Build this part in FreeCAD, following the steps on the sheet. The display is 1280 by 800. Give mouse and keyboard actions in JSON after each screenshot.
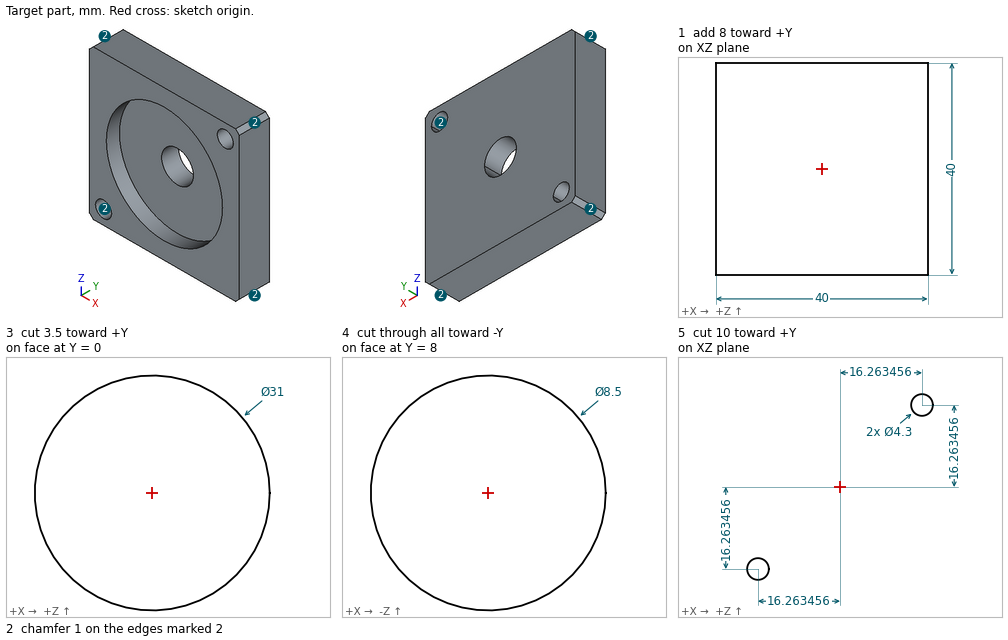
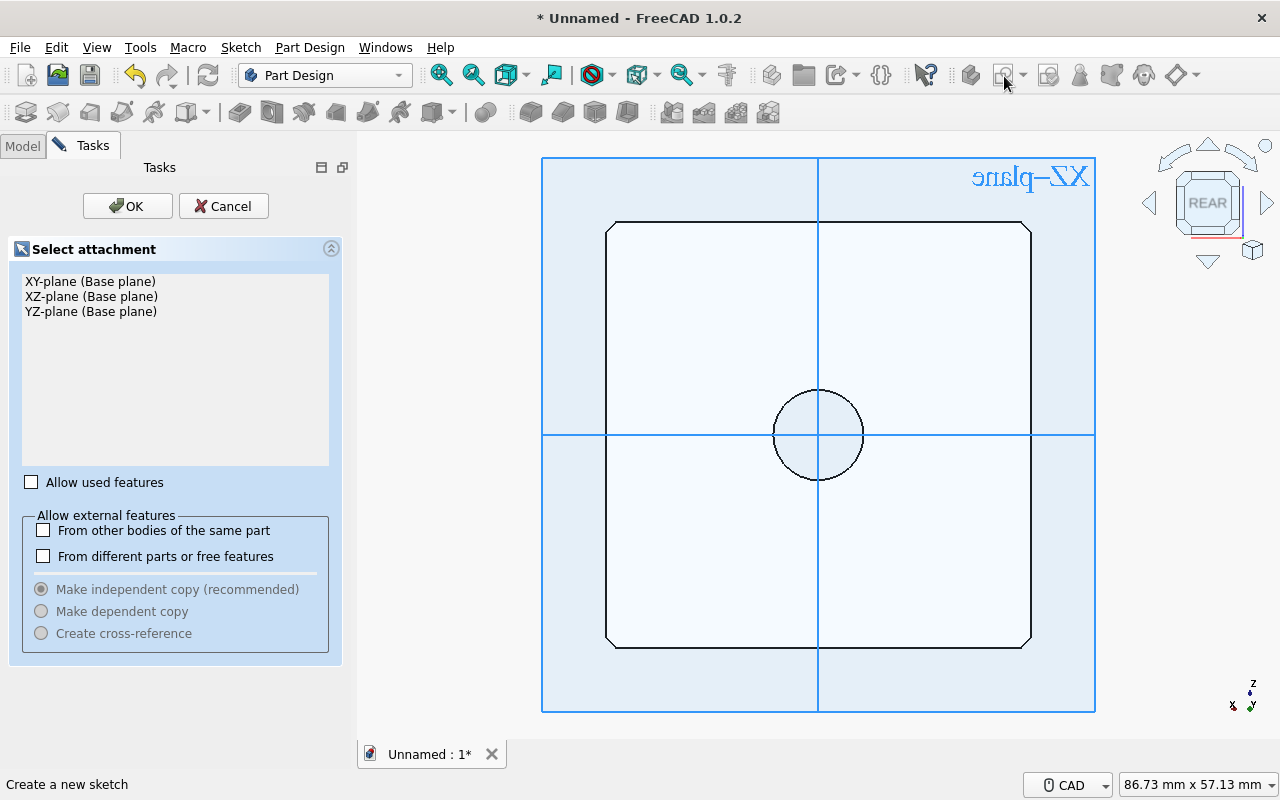
{"action": "left_click", "coordinate": [82, 296]}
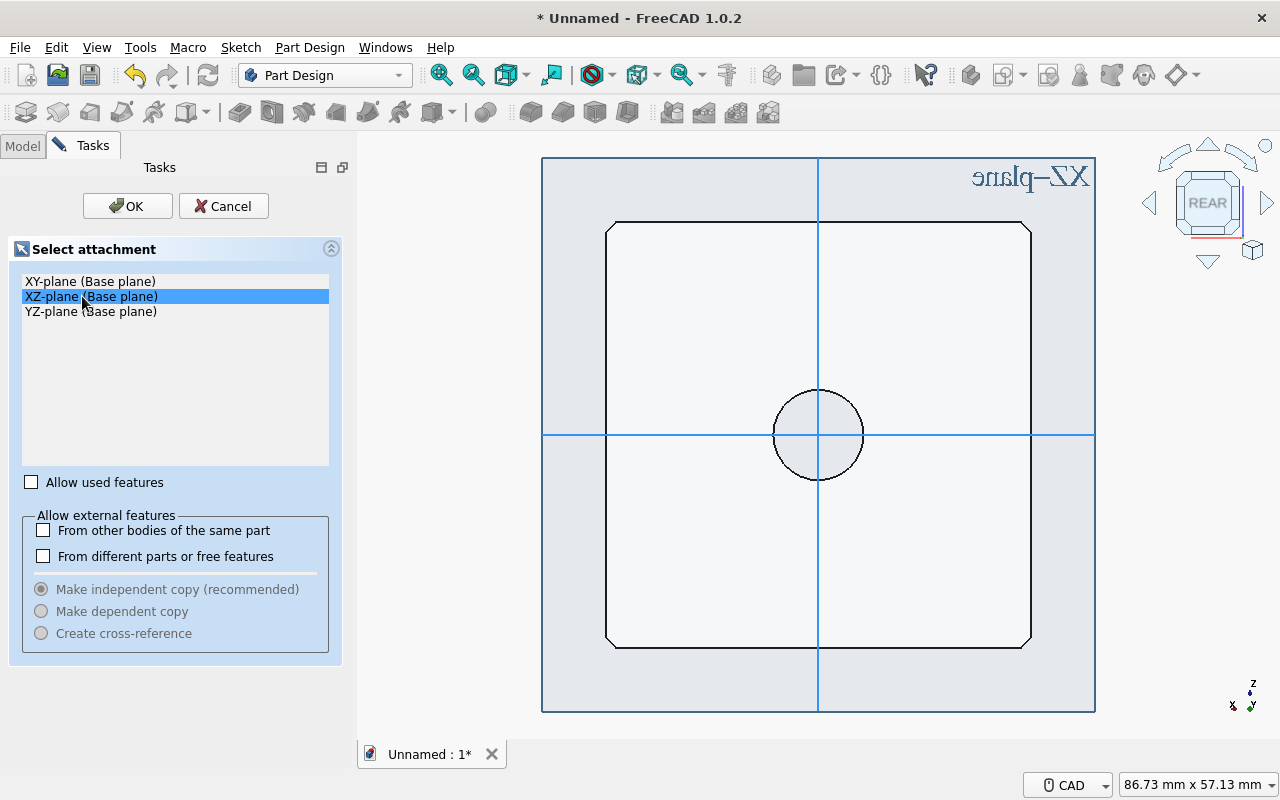
{"action": "left_click", "coordinate": [128, 206]}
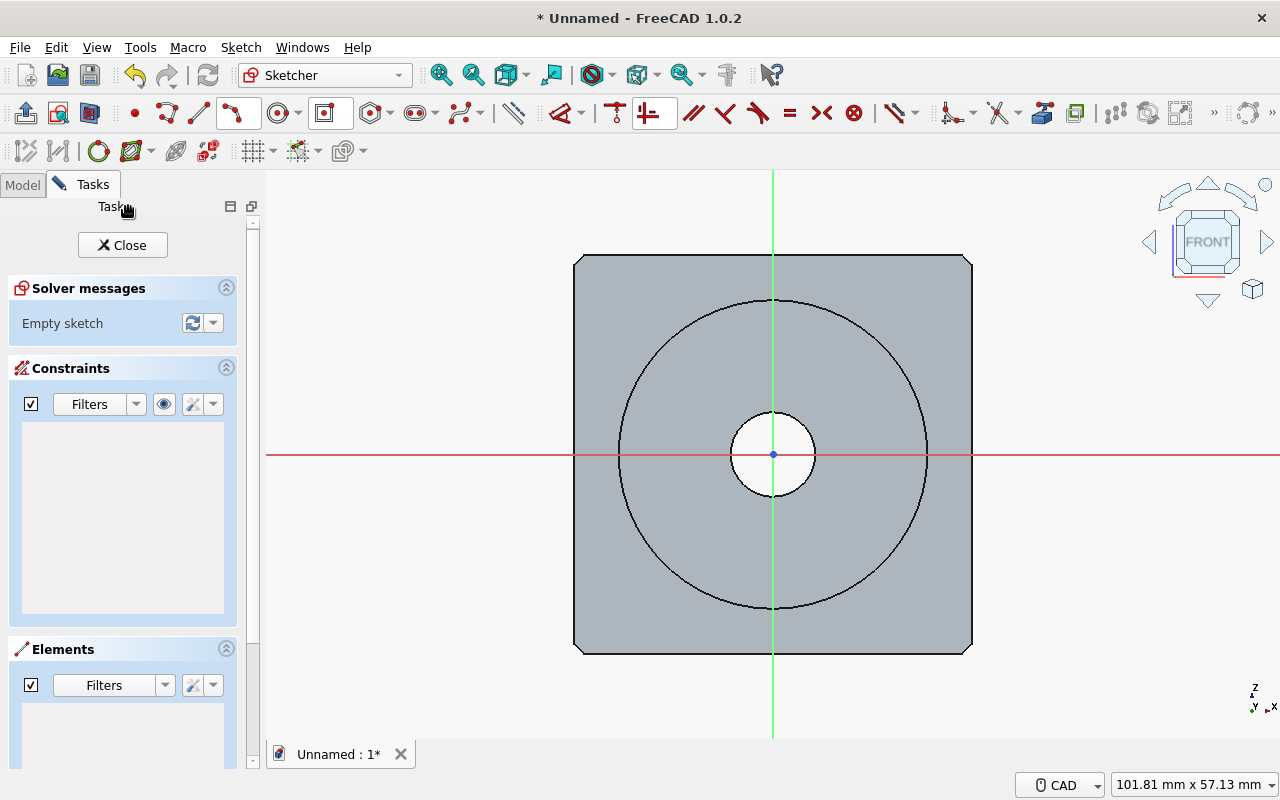
{"action": "left_click", "coordinate": [278, 114]}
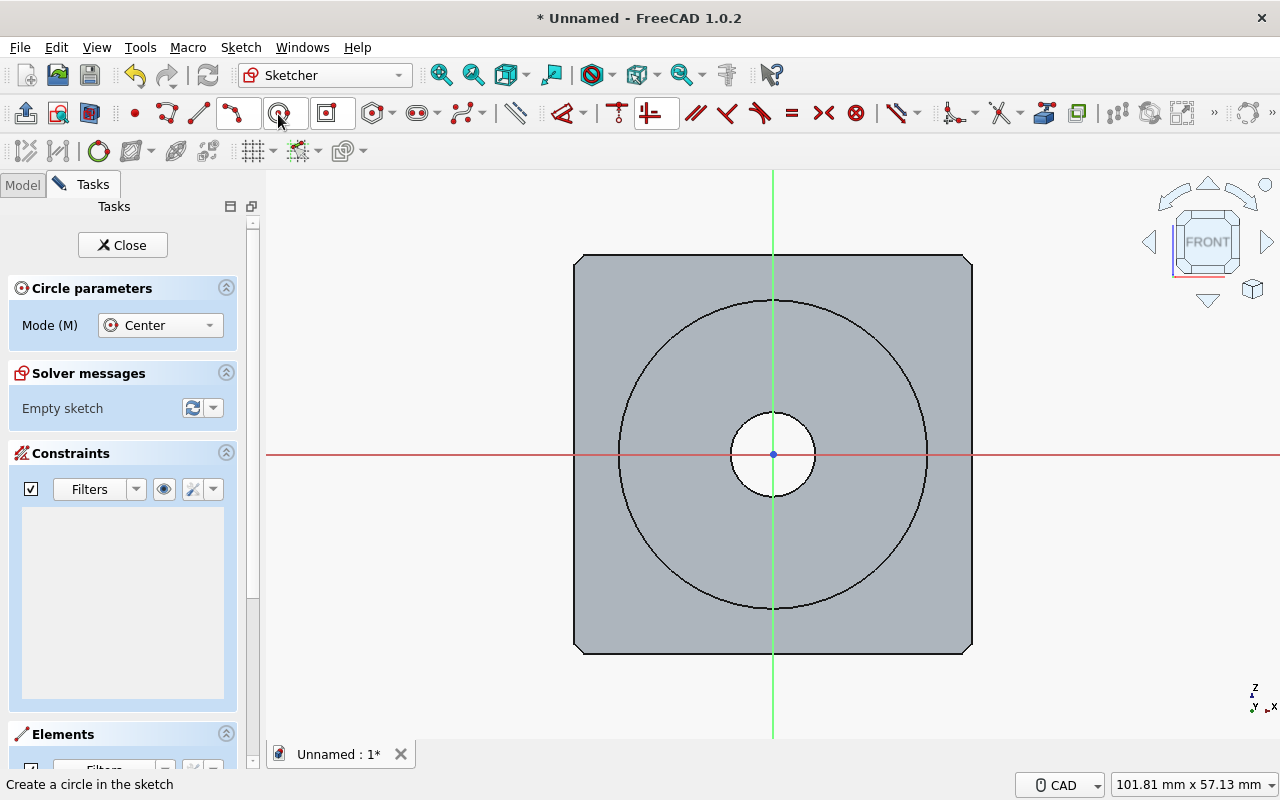
{"action": "left_click", "coordinate": [935, 293]}
{"action": "left_click", "coordinate": [950, 277]}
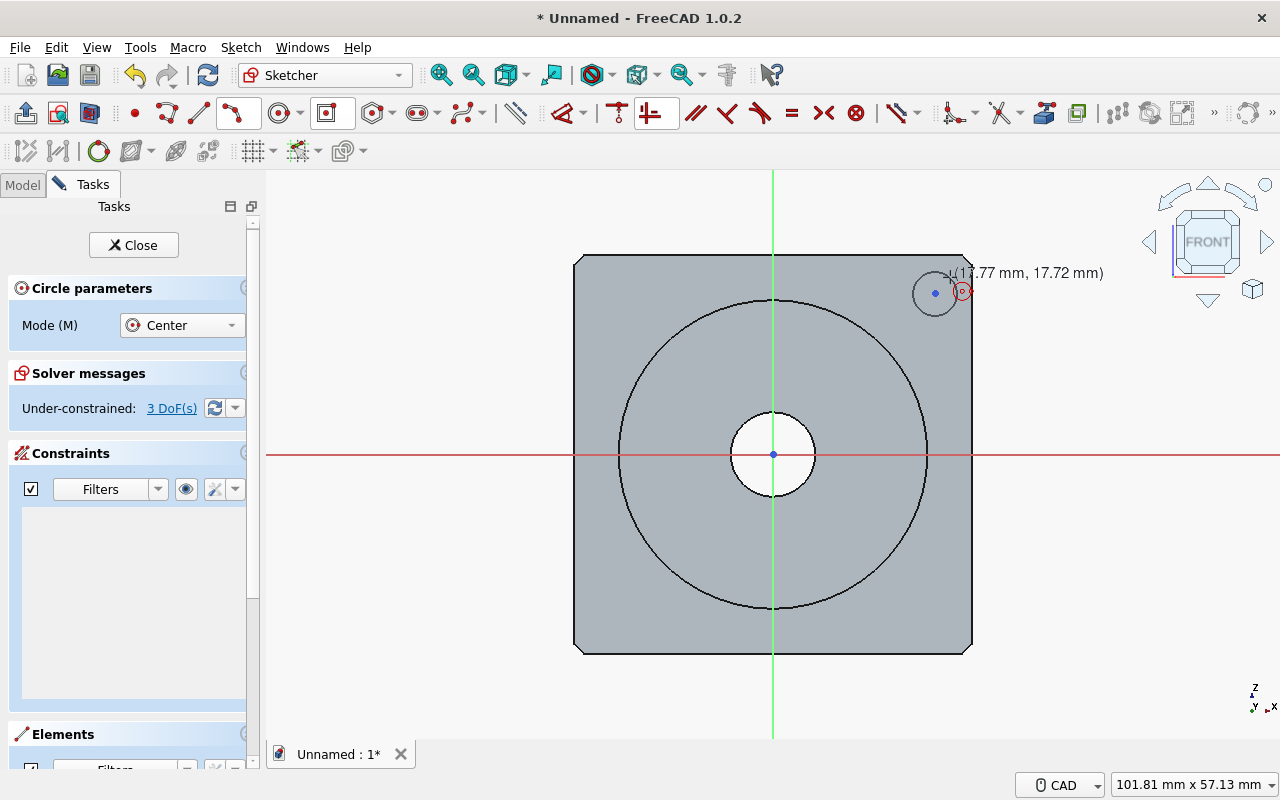
{"action": "left_click", "coordinate": [611, 616]}
{"action": "left_click", "coordinate": [626, 601]}
{"action": "key", "text": "Escape"}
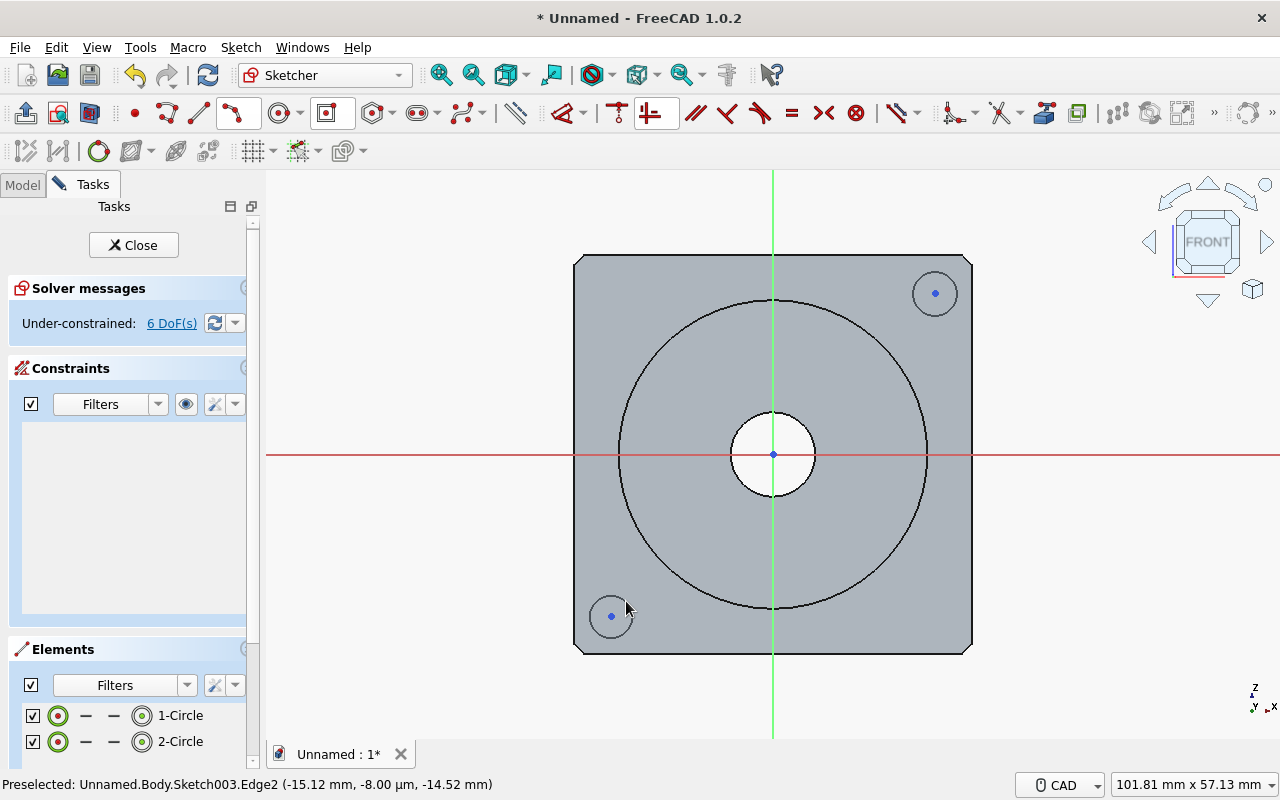
{"action": "left_click", "coordinate": [950, 278]}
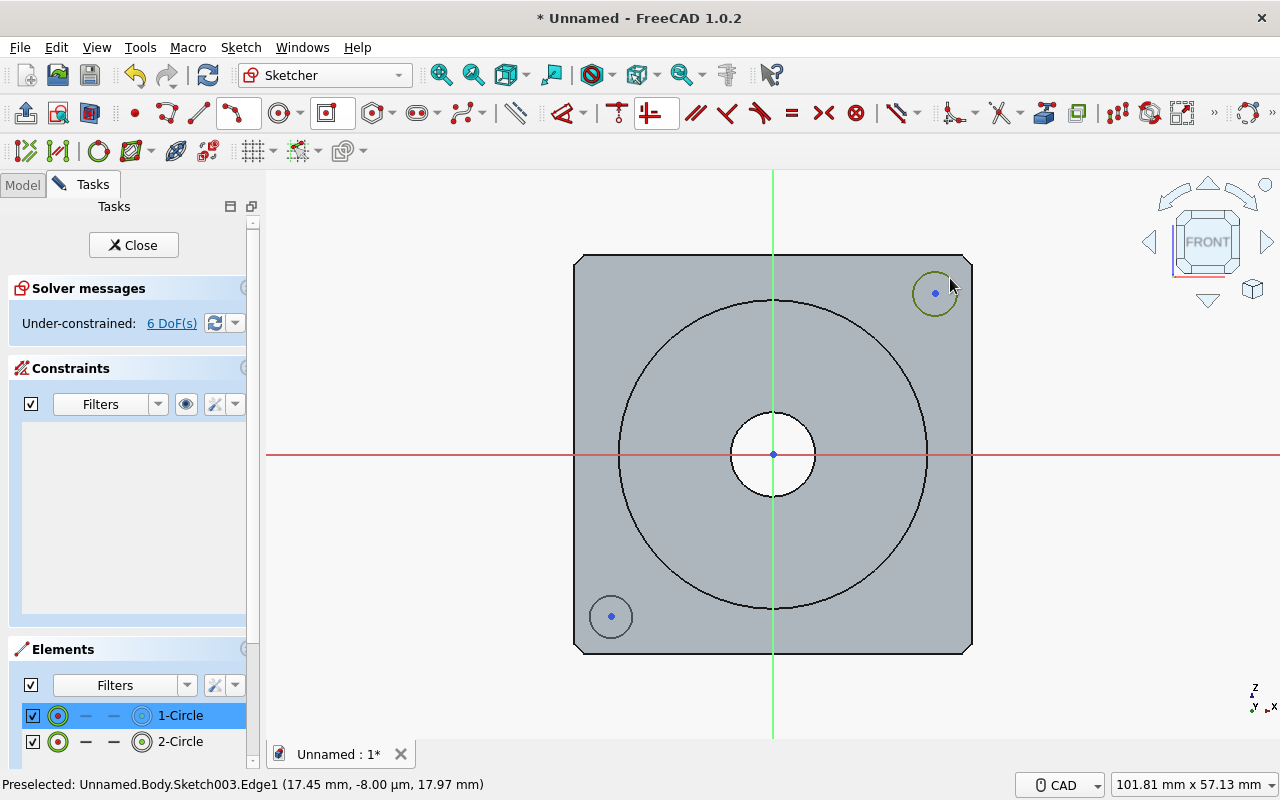
{"action": "left_click", "coordinate": [626, 602]}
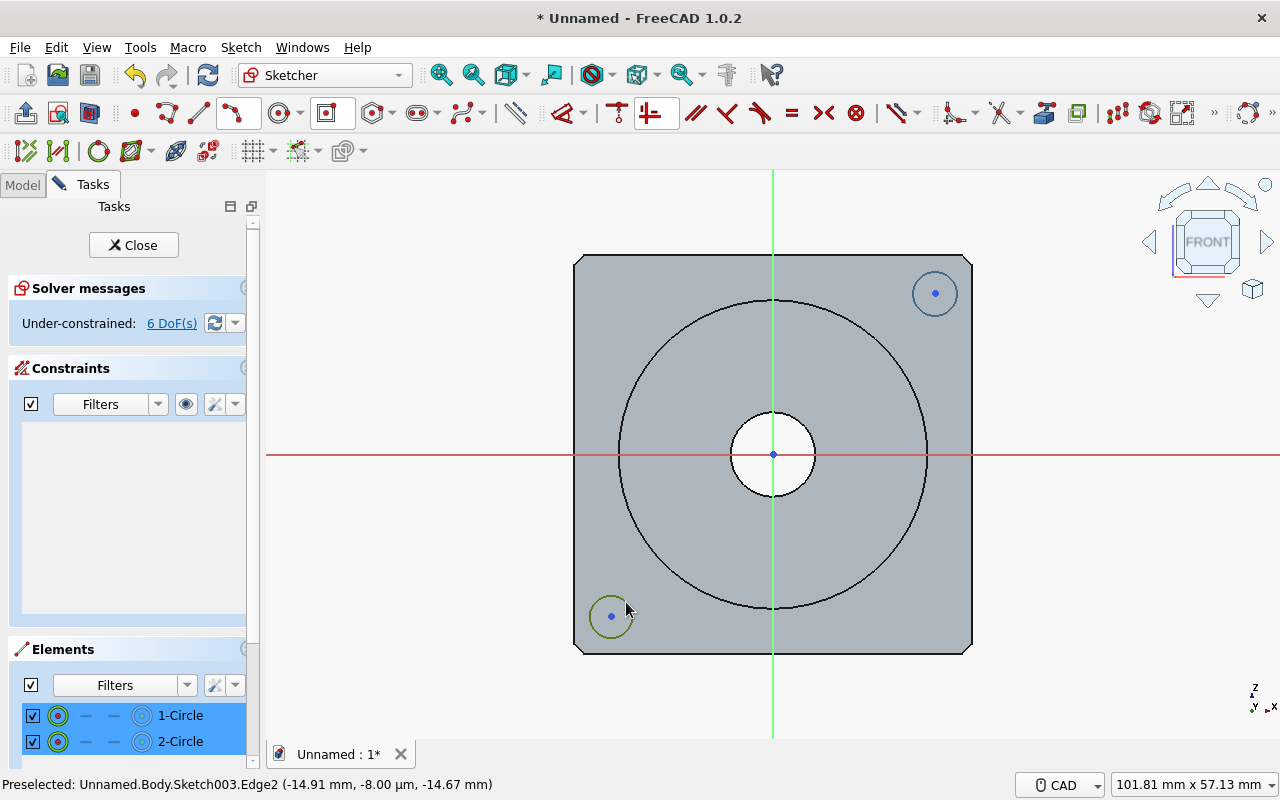
{"action": "left_click", "coordinate": [792, 114]}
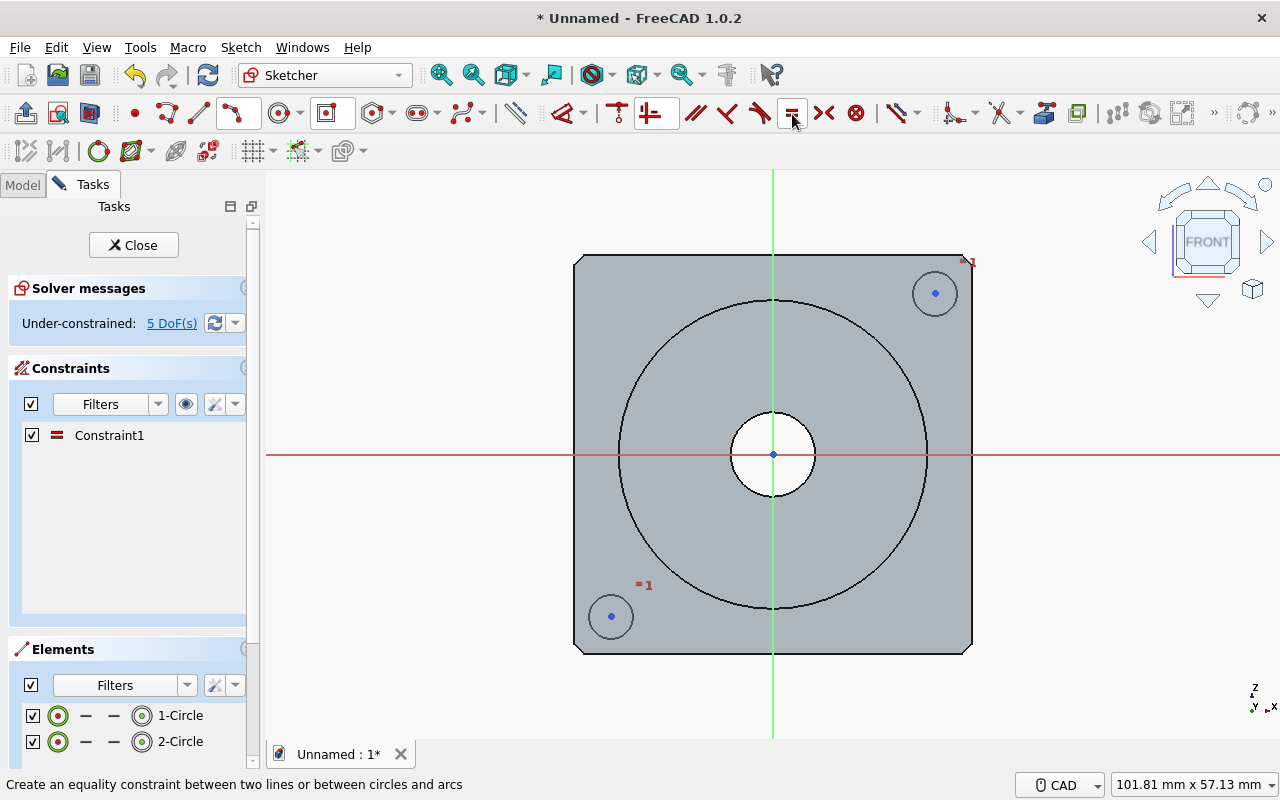
{"action": "left_click", "coordinate": [562, 114]}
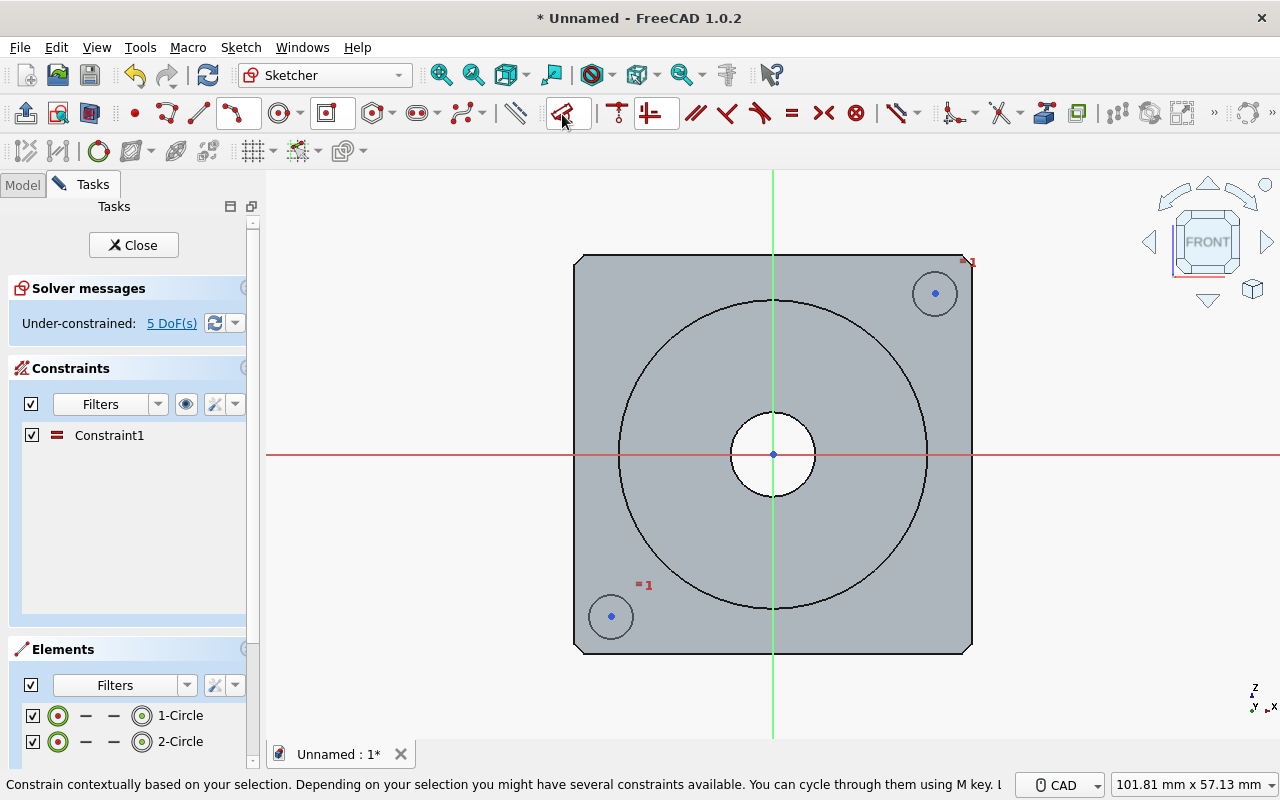
{"action": "left_click", "coordinate": [950, 278]}
{"action": "left_click", "coordinate": [972, 255]}